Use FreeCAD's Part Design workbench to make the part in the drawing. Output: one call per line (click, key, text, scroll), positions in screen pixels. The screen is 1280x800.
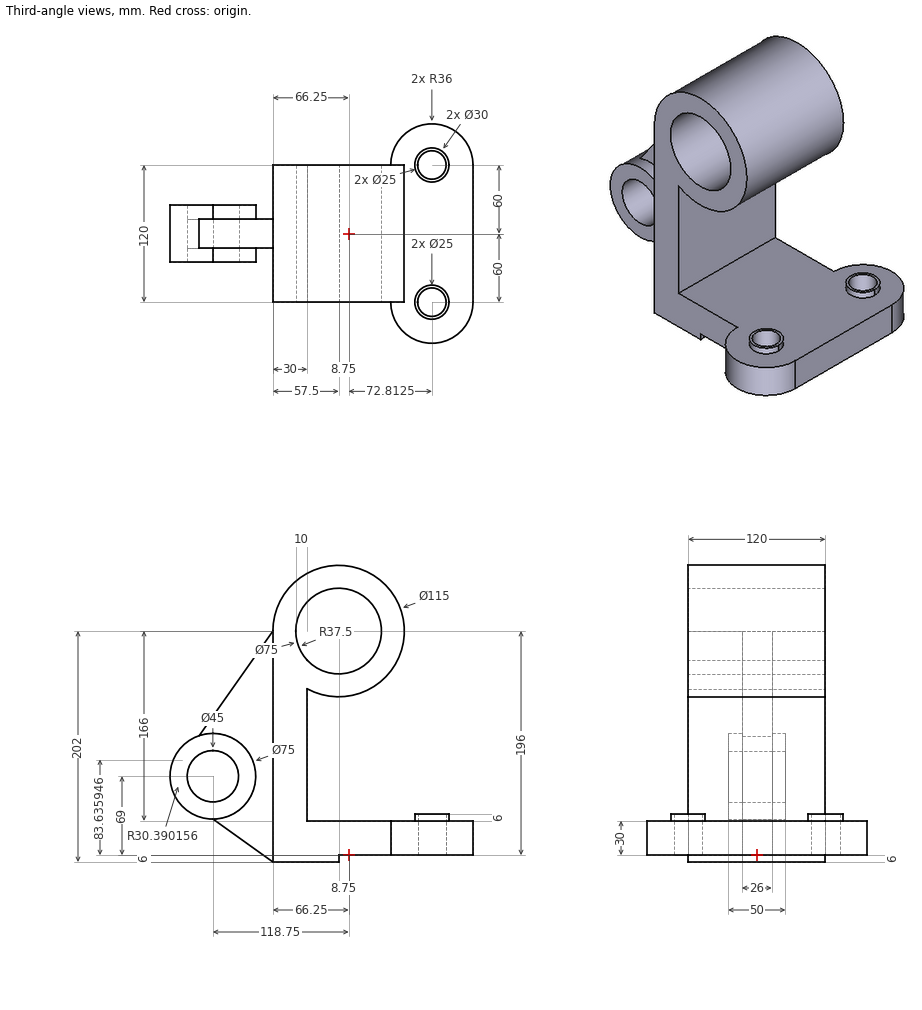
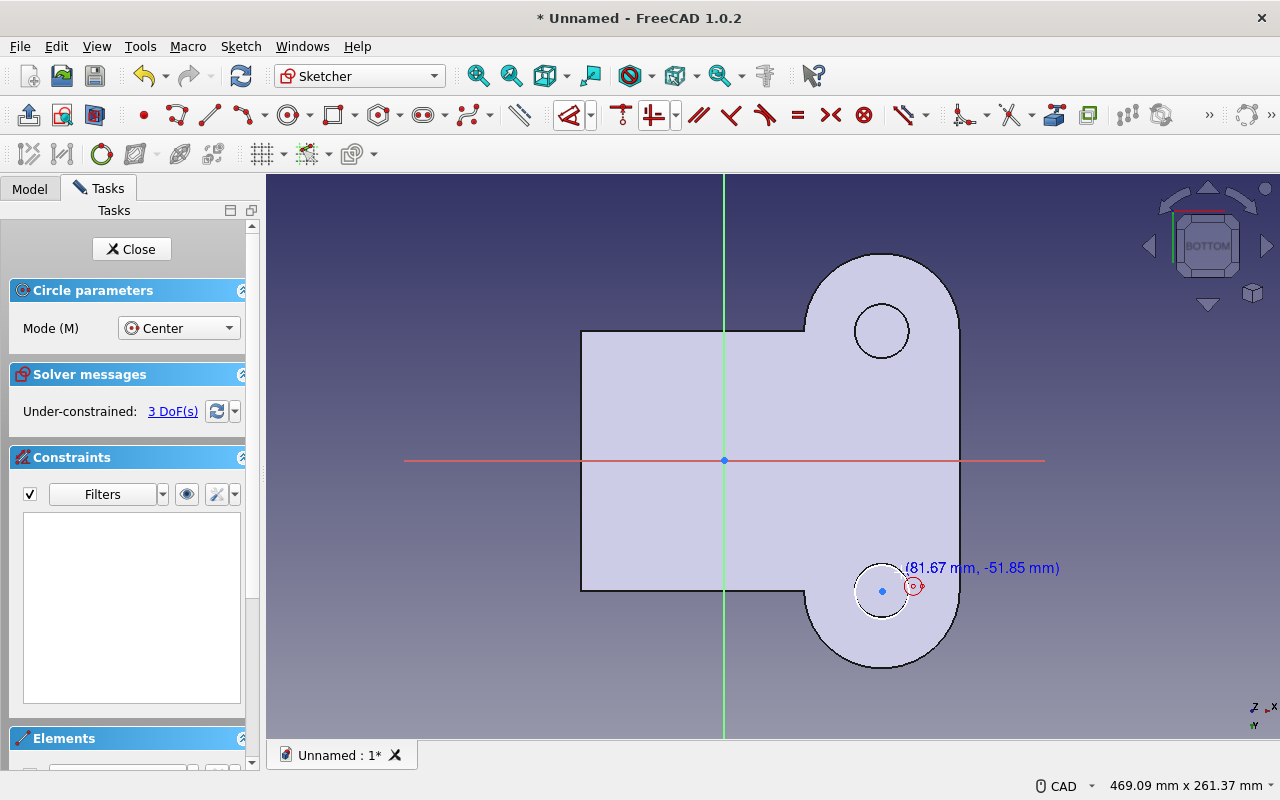
click(882, 331)
click(901, 312)
key(Escape)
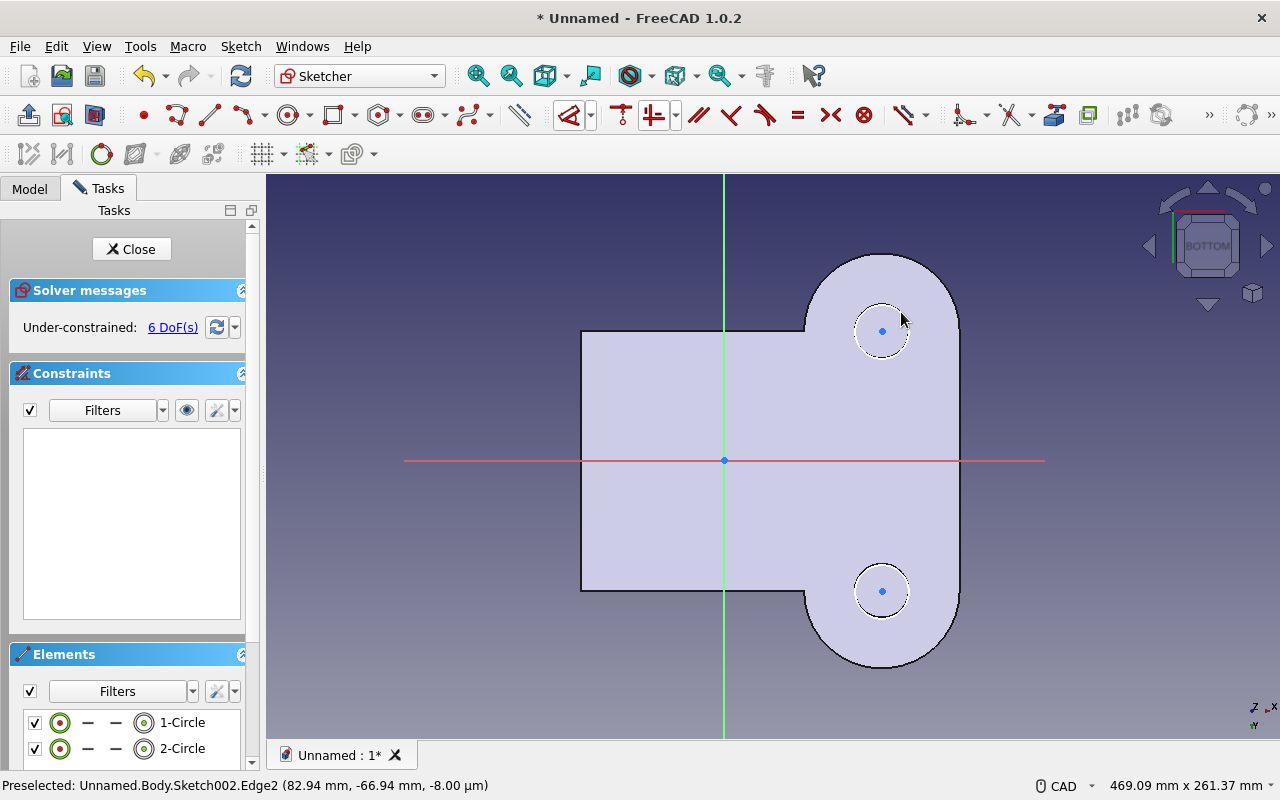
click(901, 573)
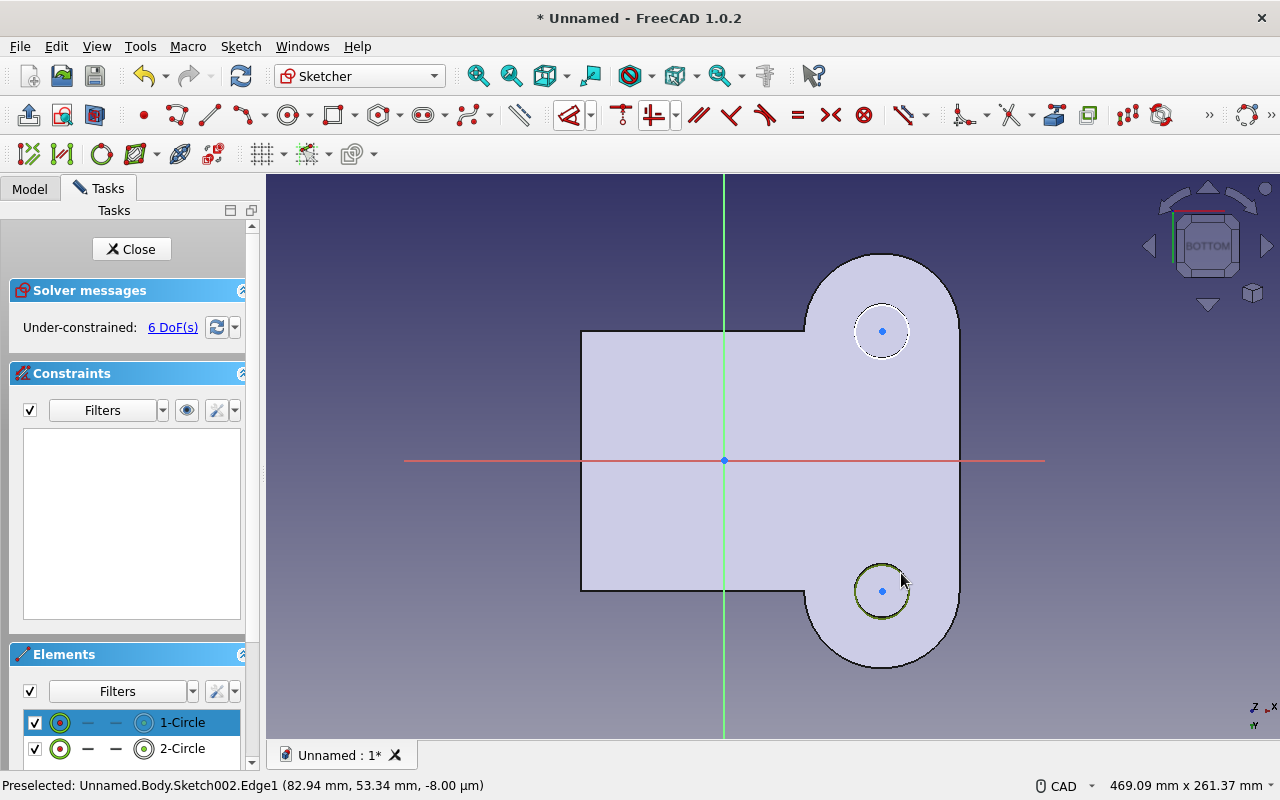
click(901, 313)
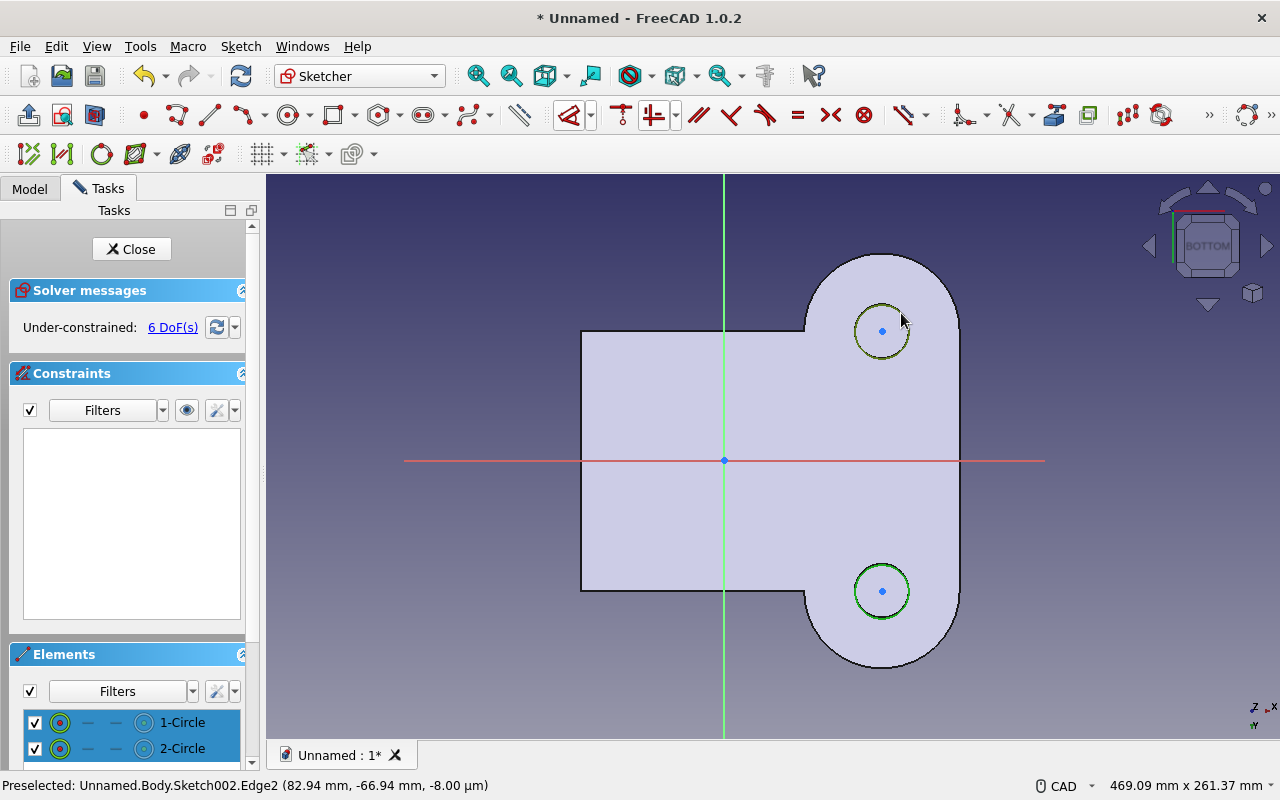
key(e)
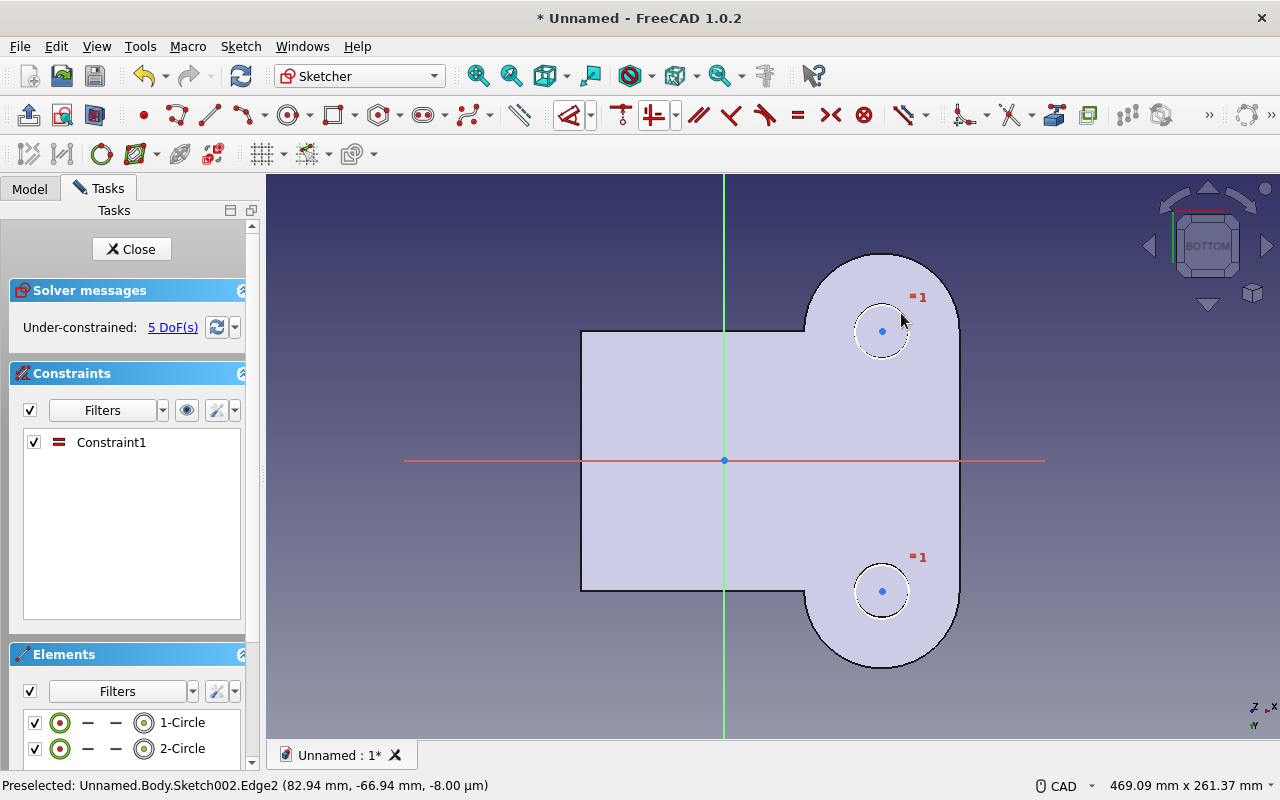
click(882, 592)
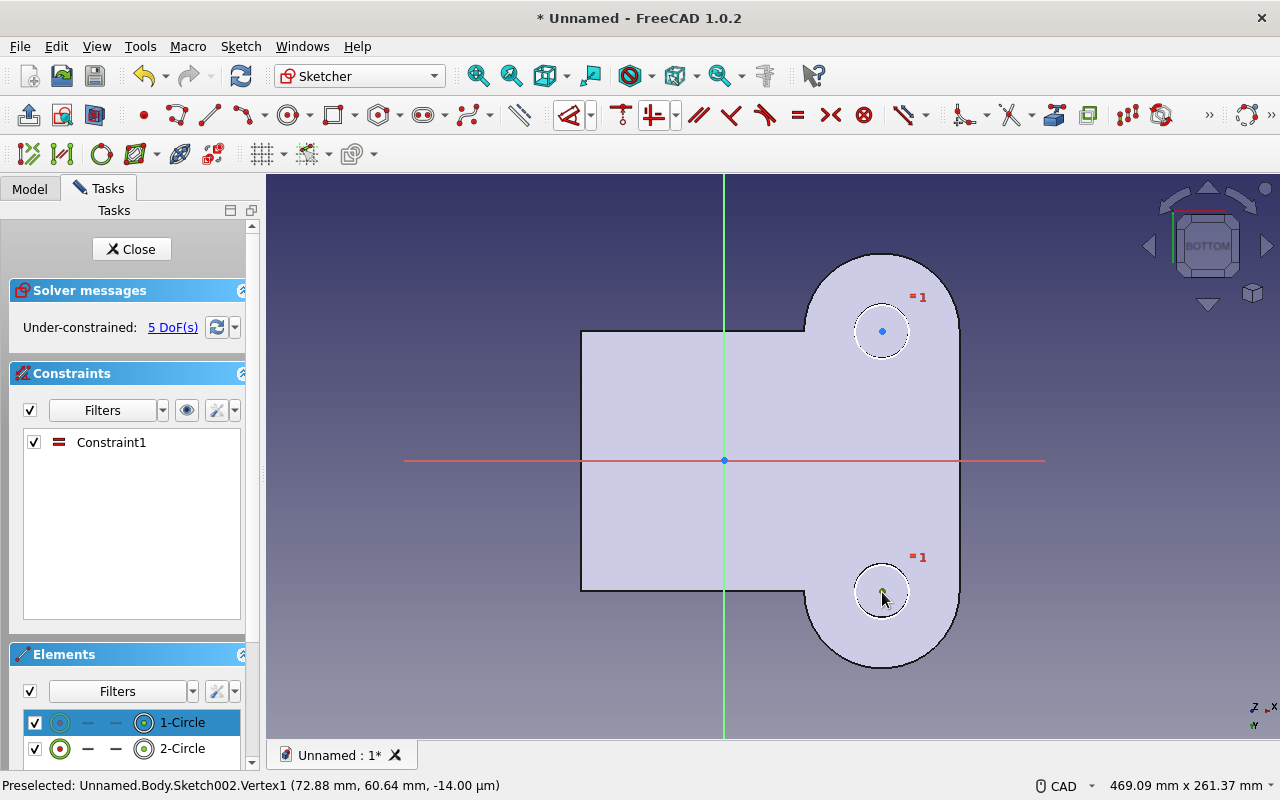
click(882, 332)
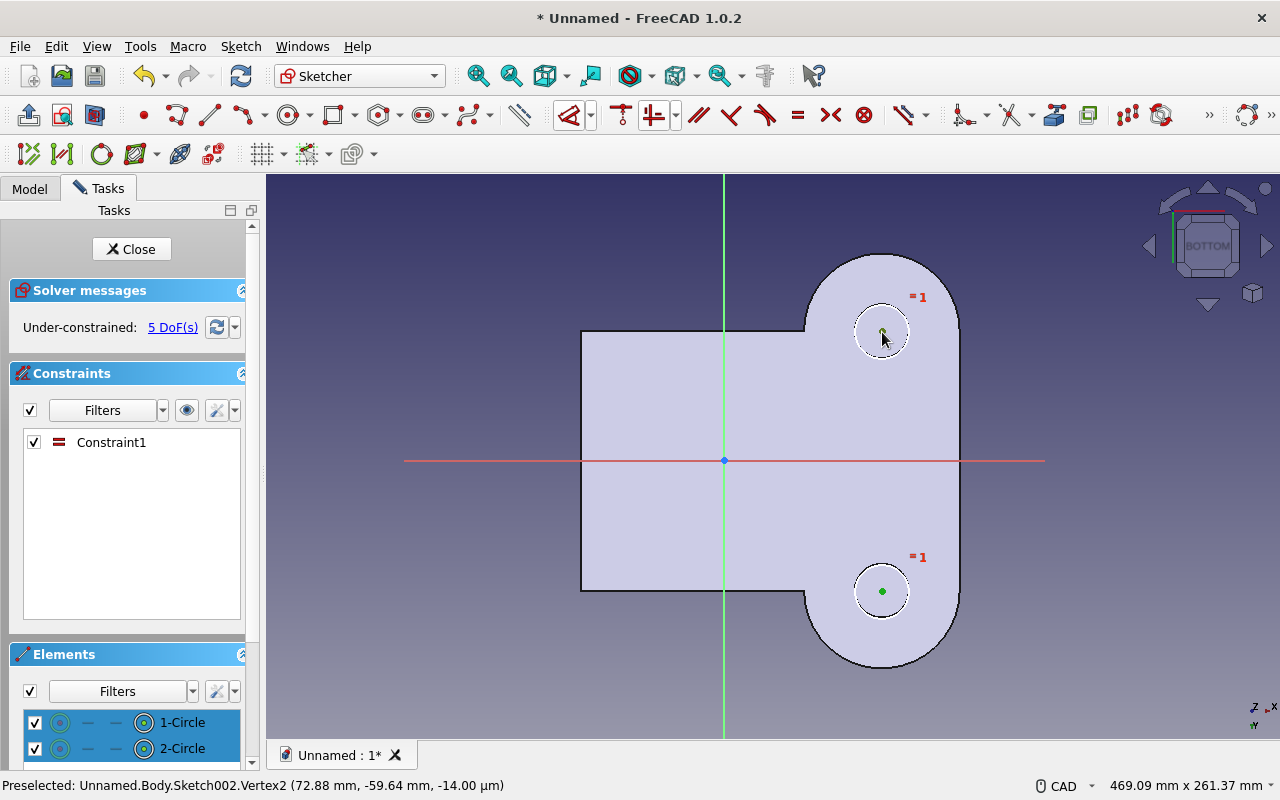
click(676, 116)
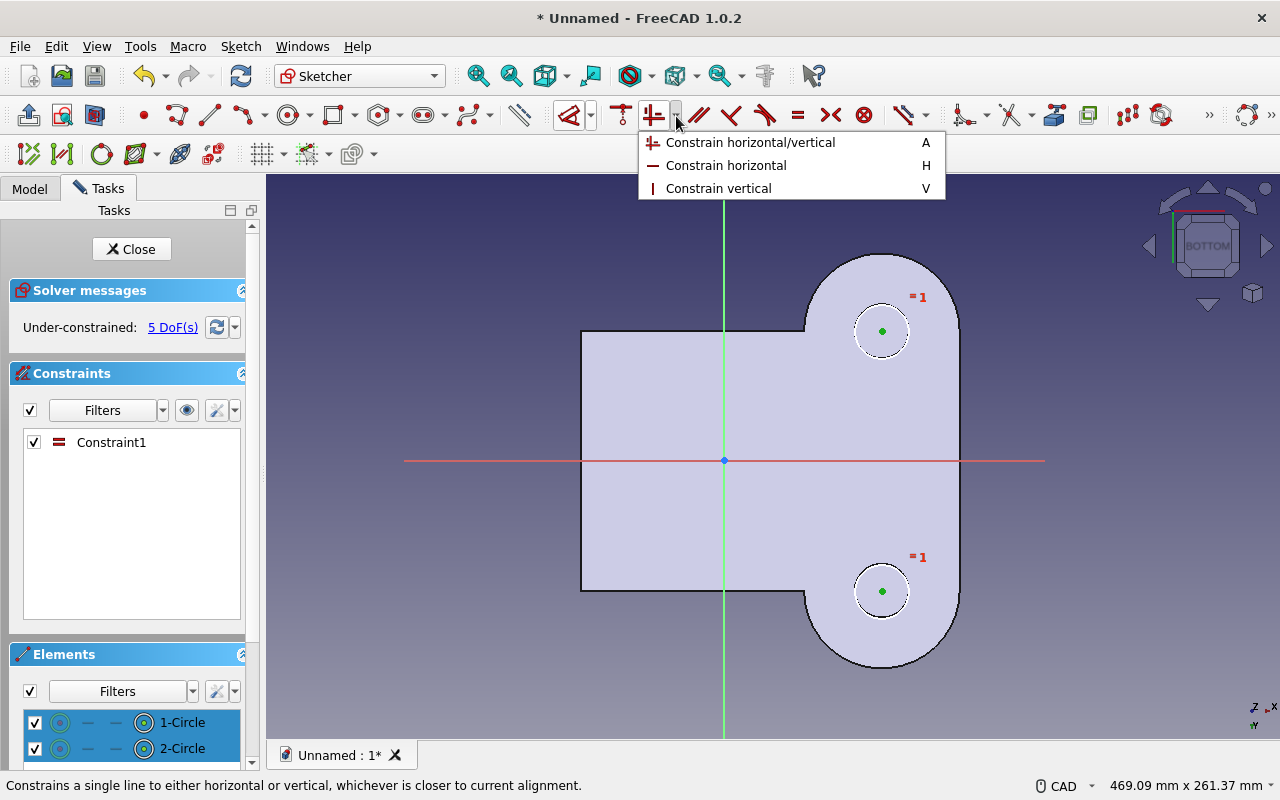
click(792, 188)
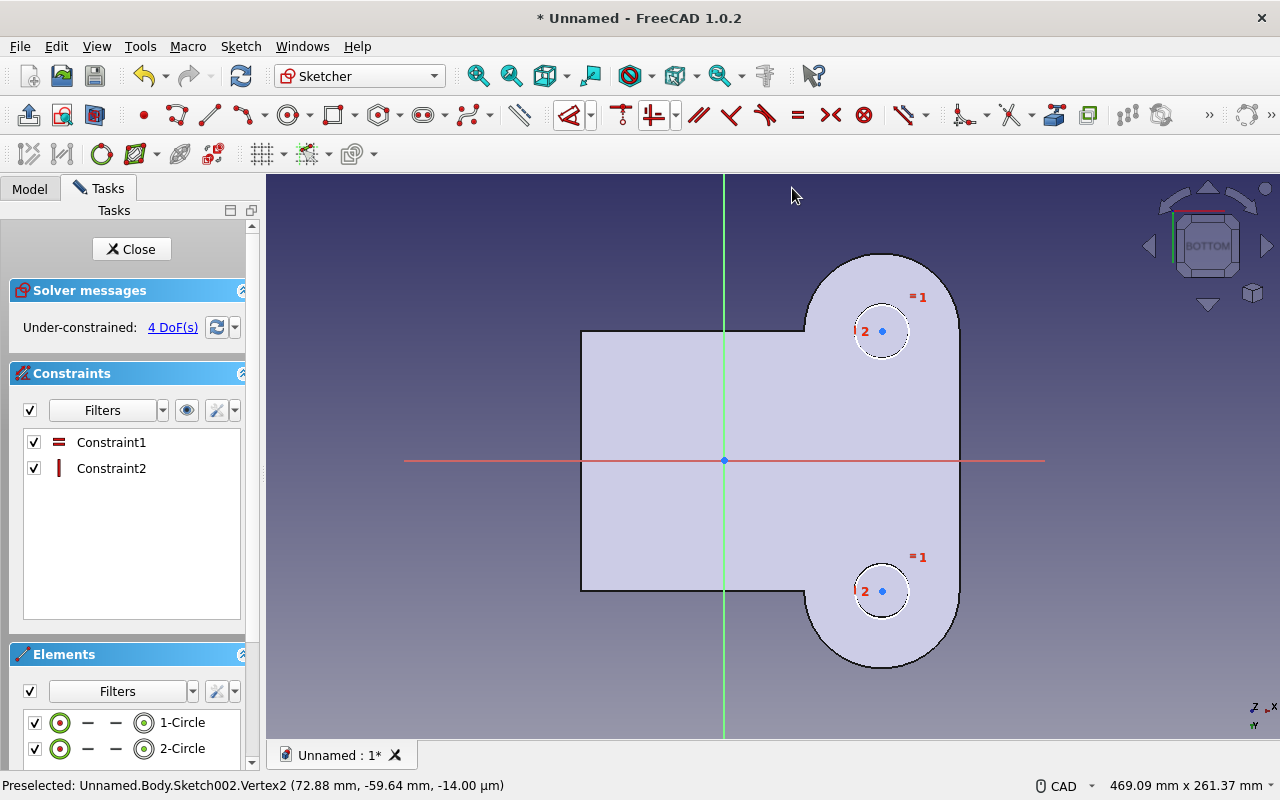
click(901, 573)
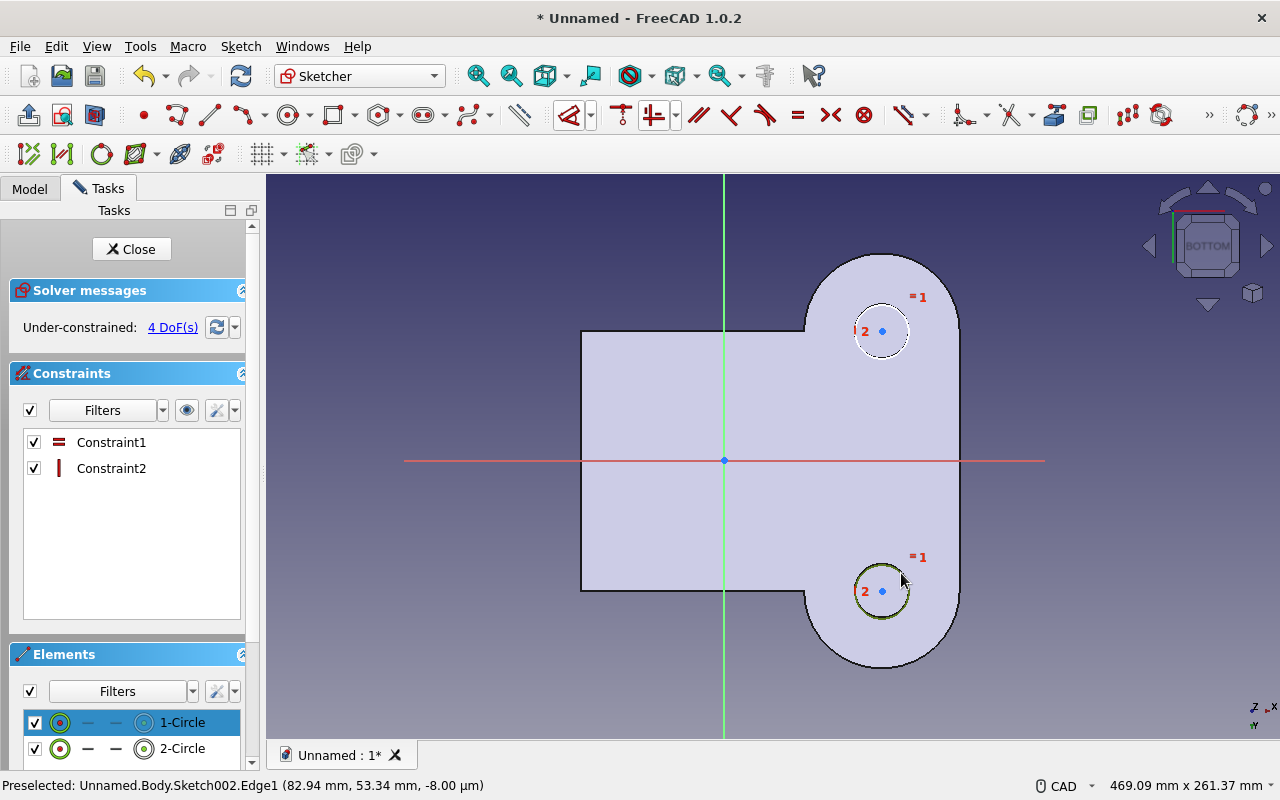
click(590, 116)